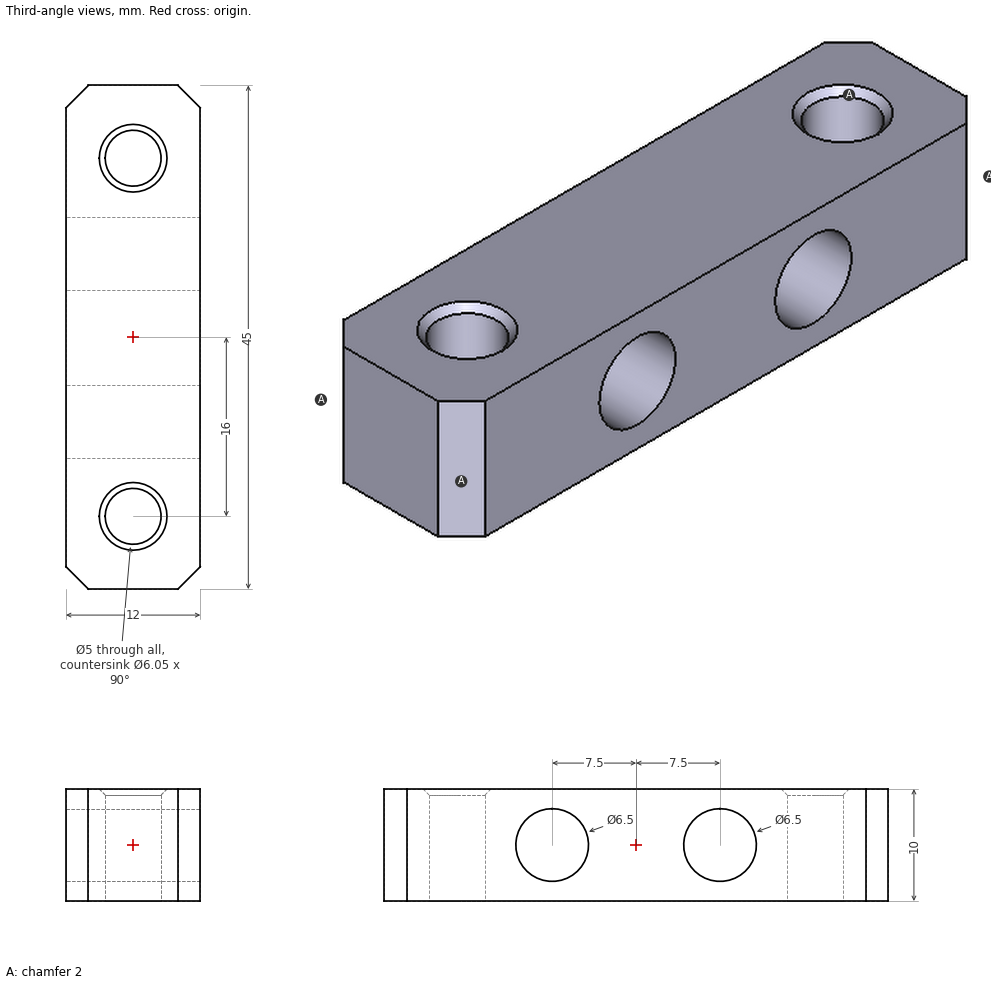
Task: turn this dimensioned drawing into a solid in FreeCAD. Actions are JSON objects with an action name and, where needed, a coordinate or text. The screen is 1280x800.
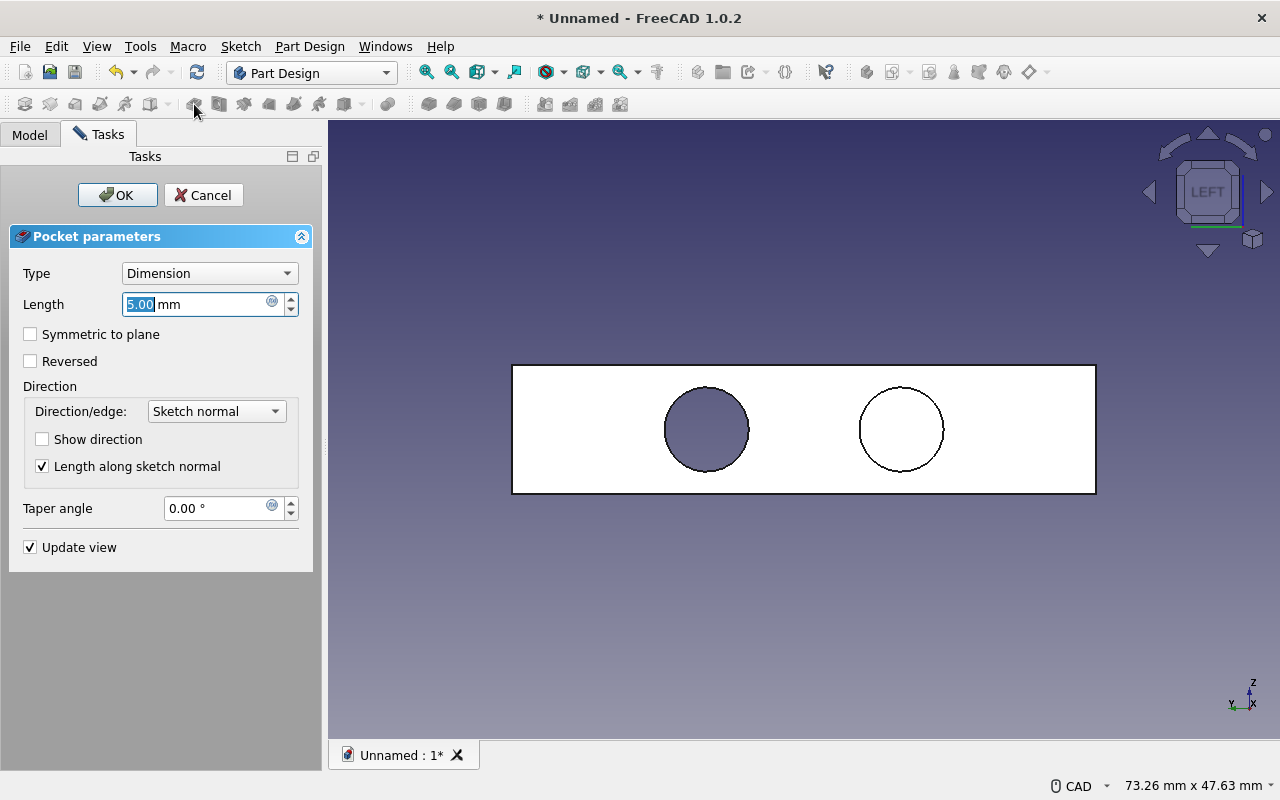
{"action": "left_click", "coordinate": [210, 274]}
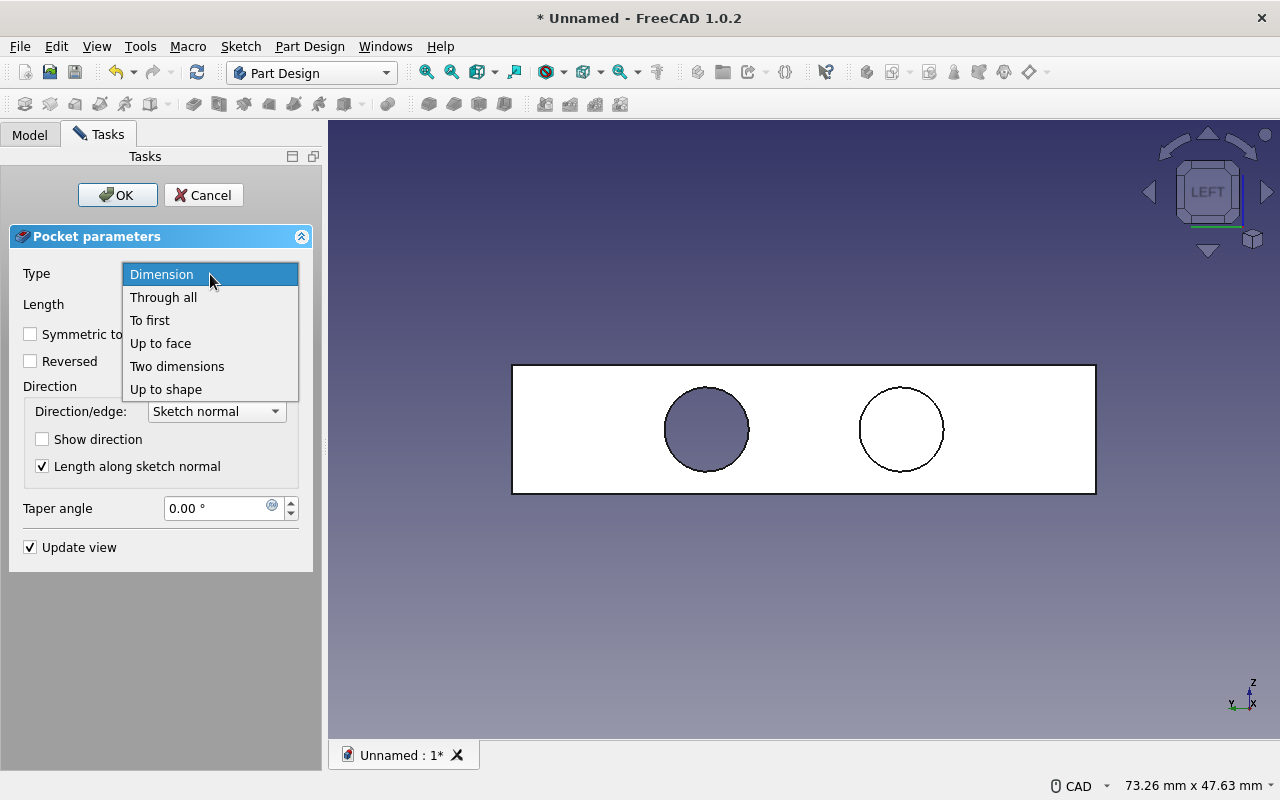
{"action": "left_click", "coordinate": [208, 320]}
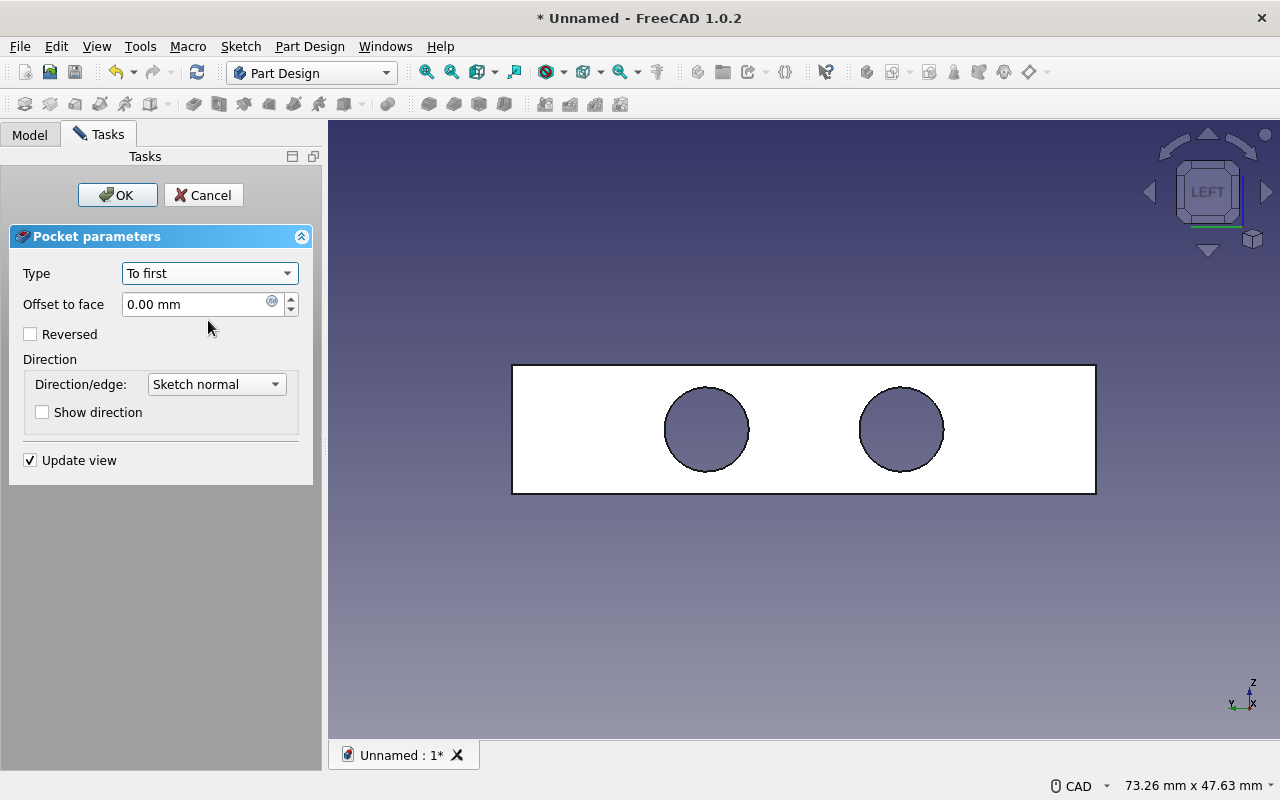
{"action": "left_click", "coordinate": [118, 195]}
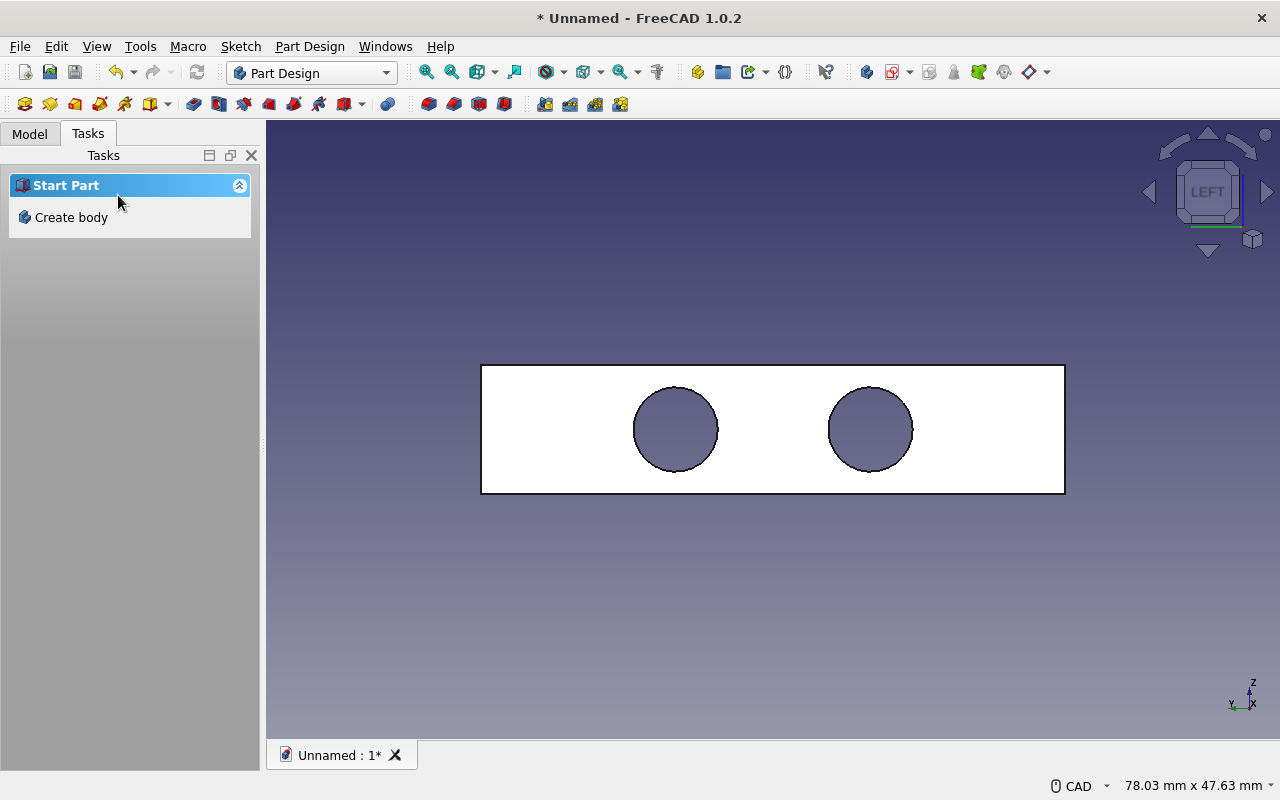
{"action": "left_click", "coordinate": [30, 134]}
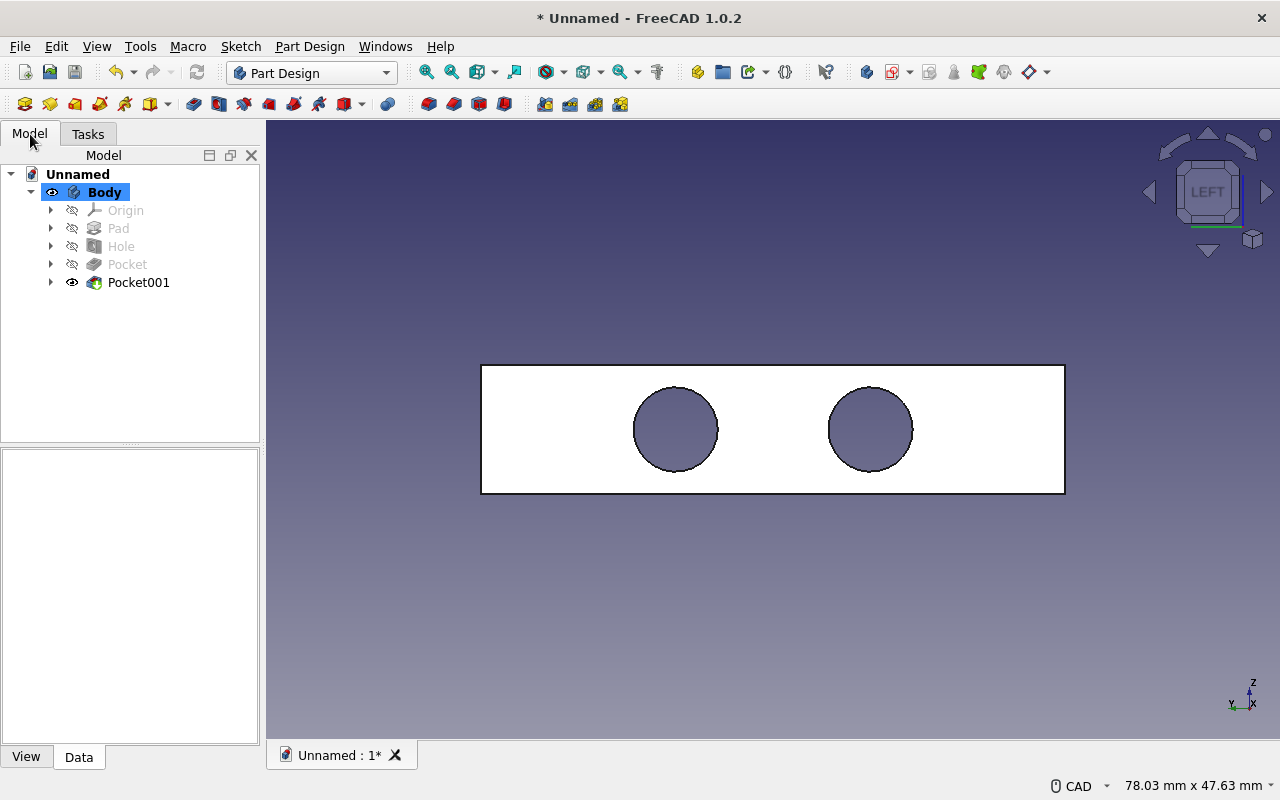
{"action": "left_click", "coordinate": [117, 246]}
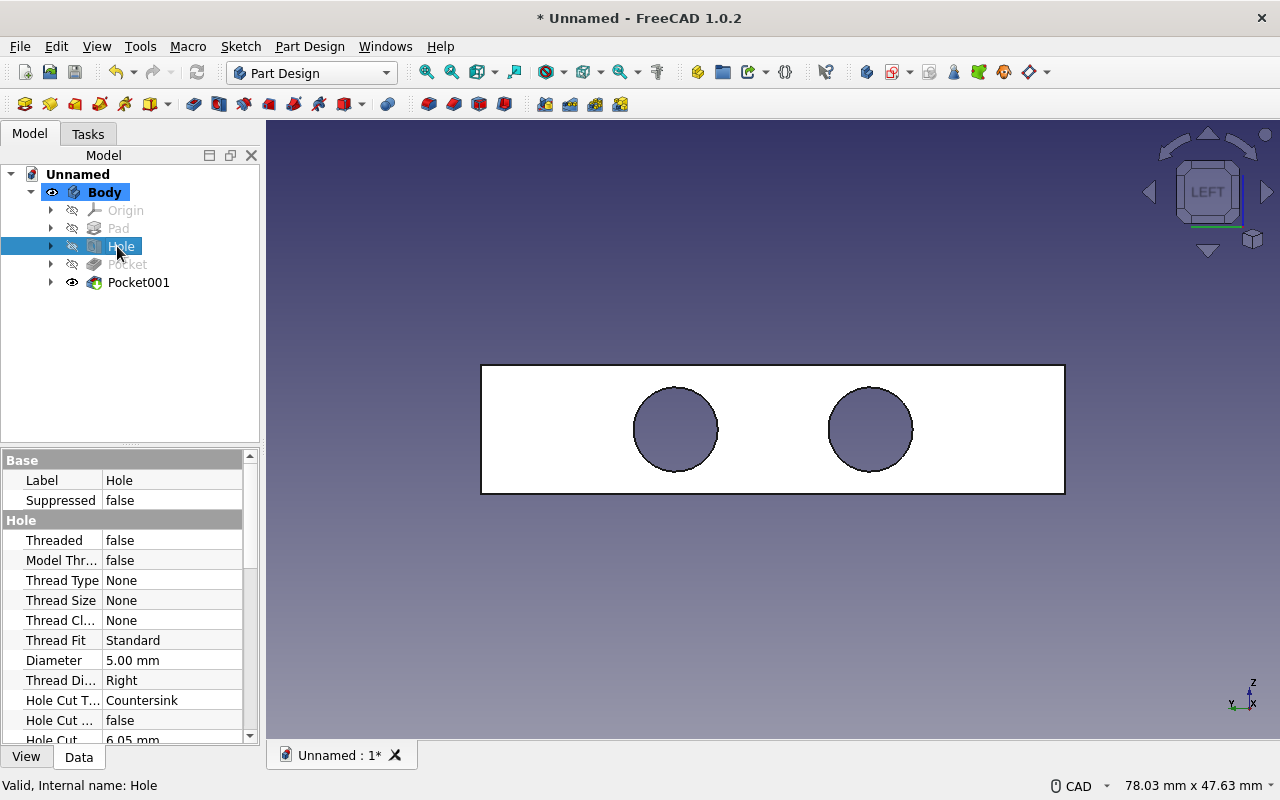
{"action": "left_click", "coordinate": [545, 104]}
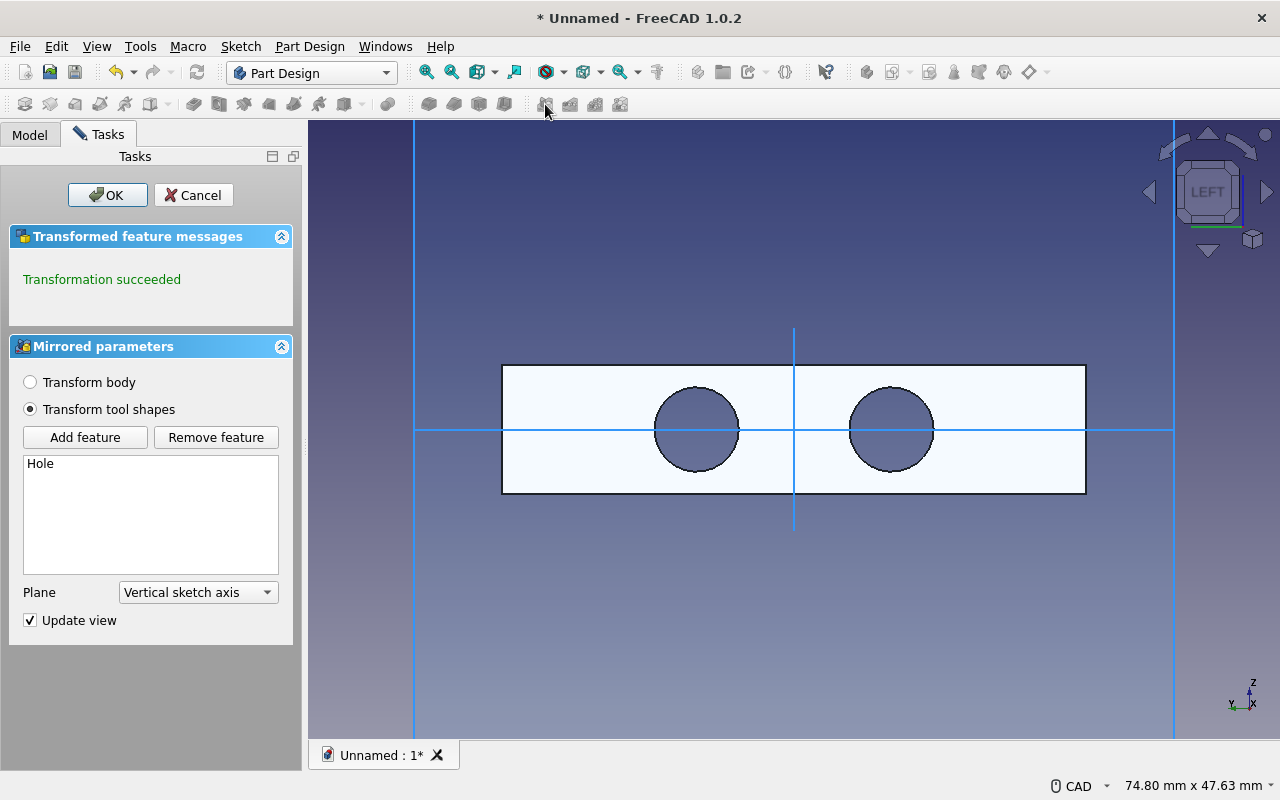
{"action": "left_click", "coordinate": [199, 592]}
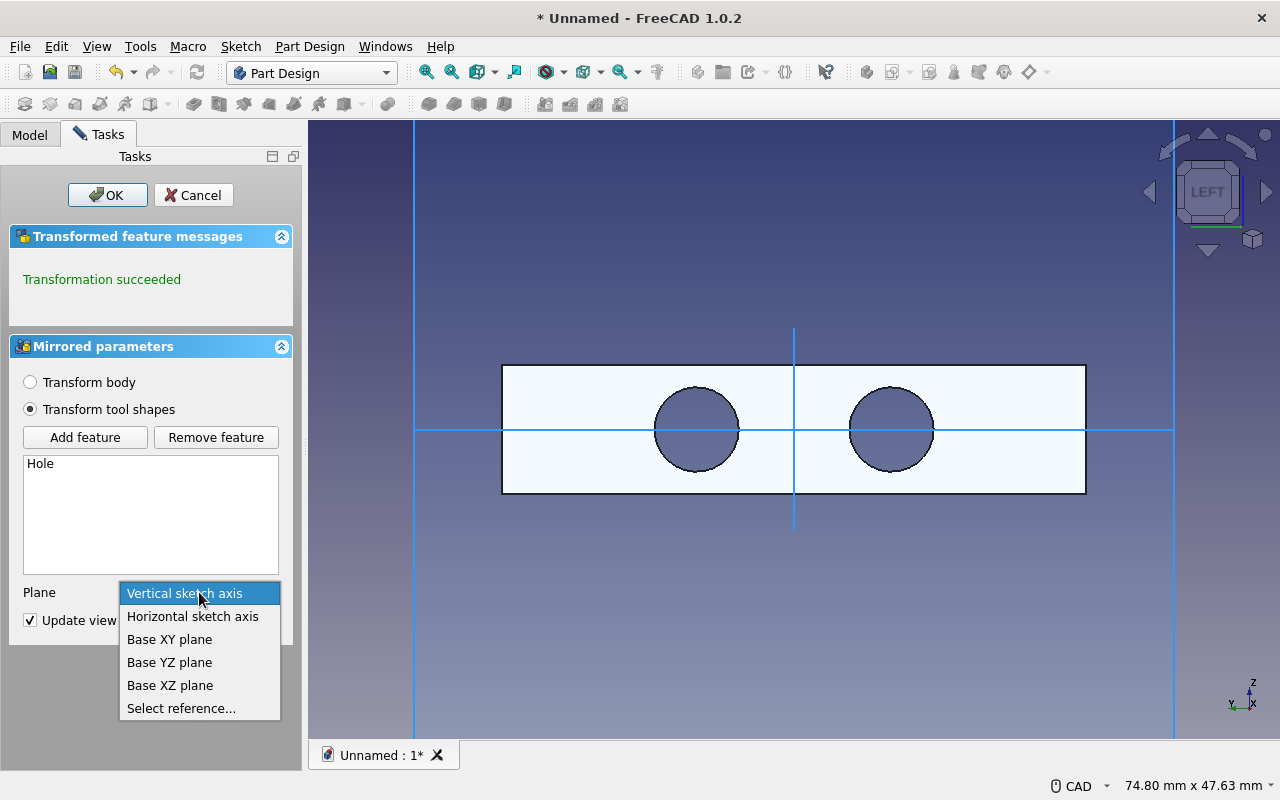
{"action": "left_click", "coordinate": [198, 686]}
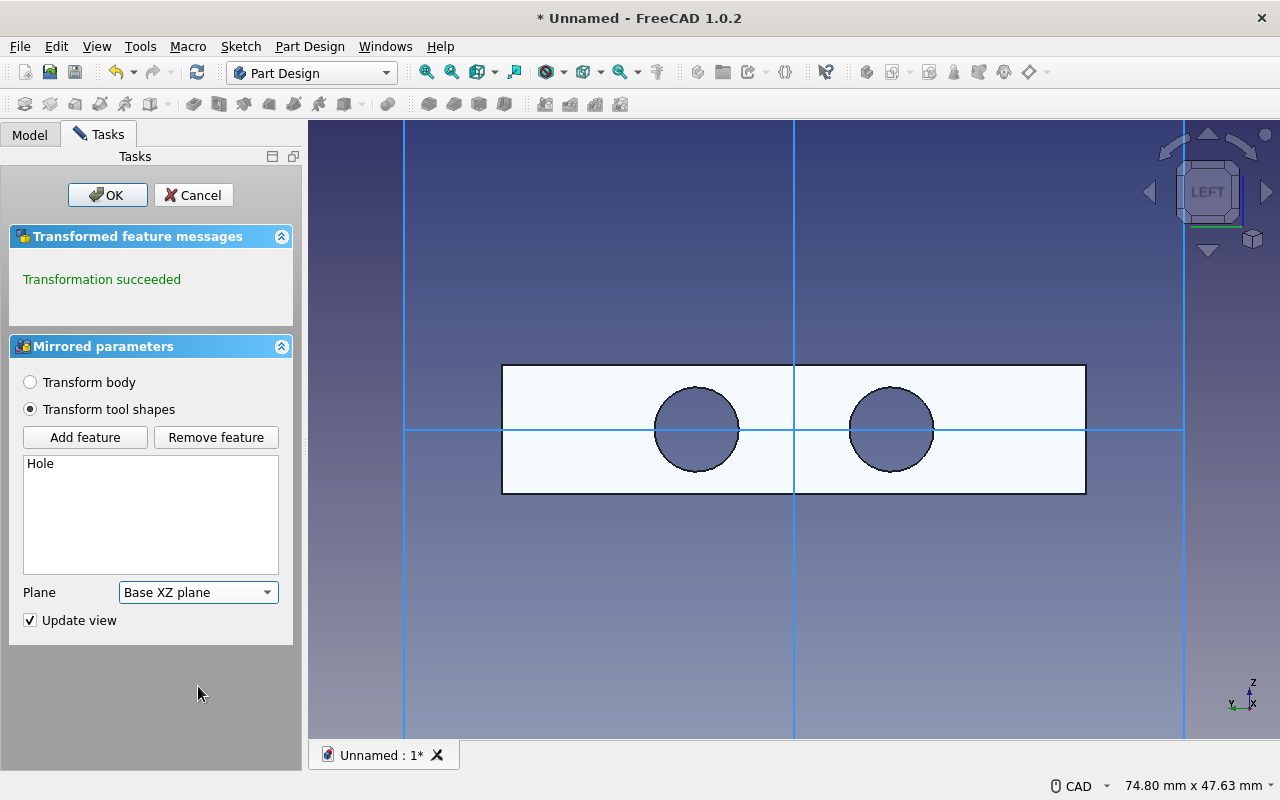
{"action": "left_click", "coordinate": [108, 195]}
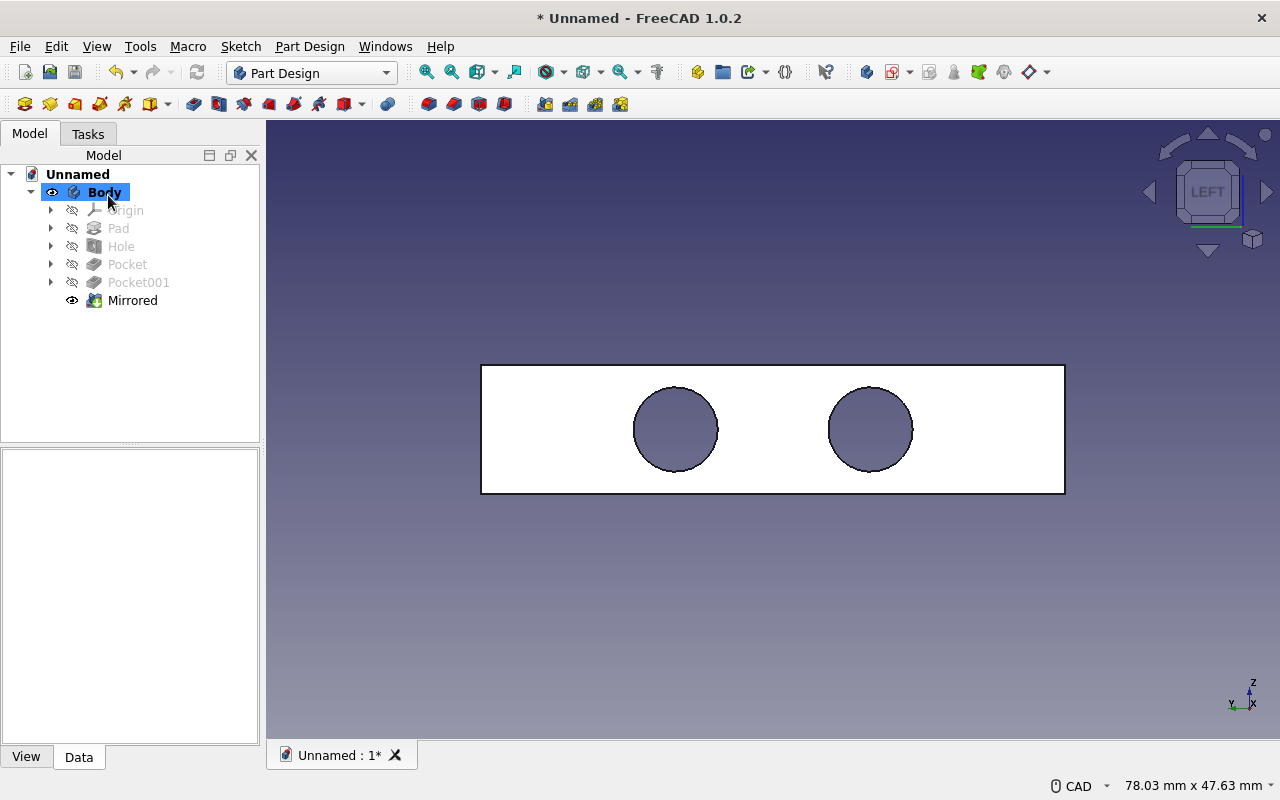
{"action": "left_click", "coordinate": [1065, 428]}